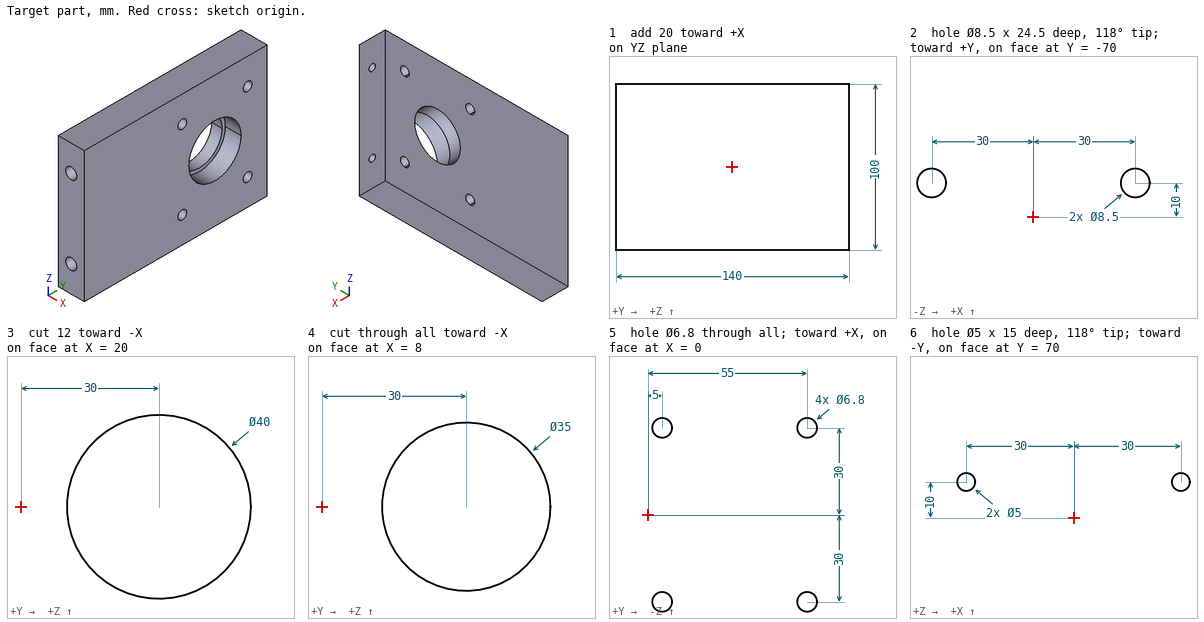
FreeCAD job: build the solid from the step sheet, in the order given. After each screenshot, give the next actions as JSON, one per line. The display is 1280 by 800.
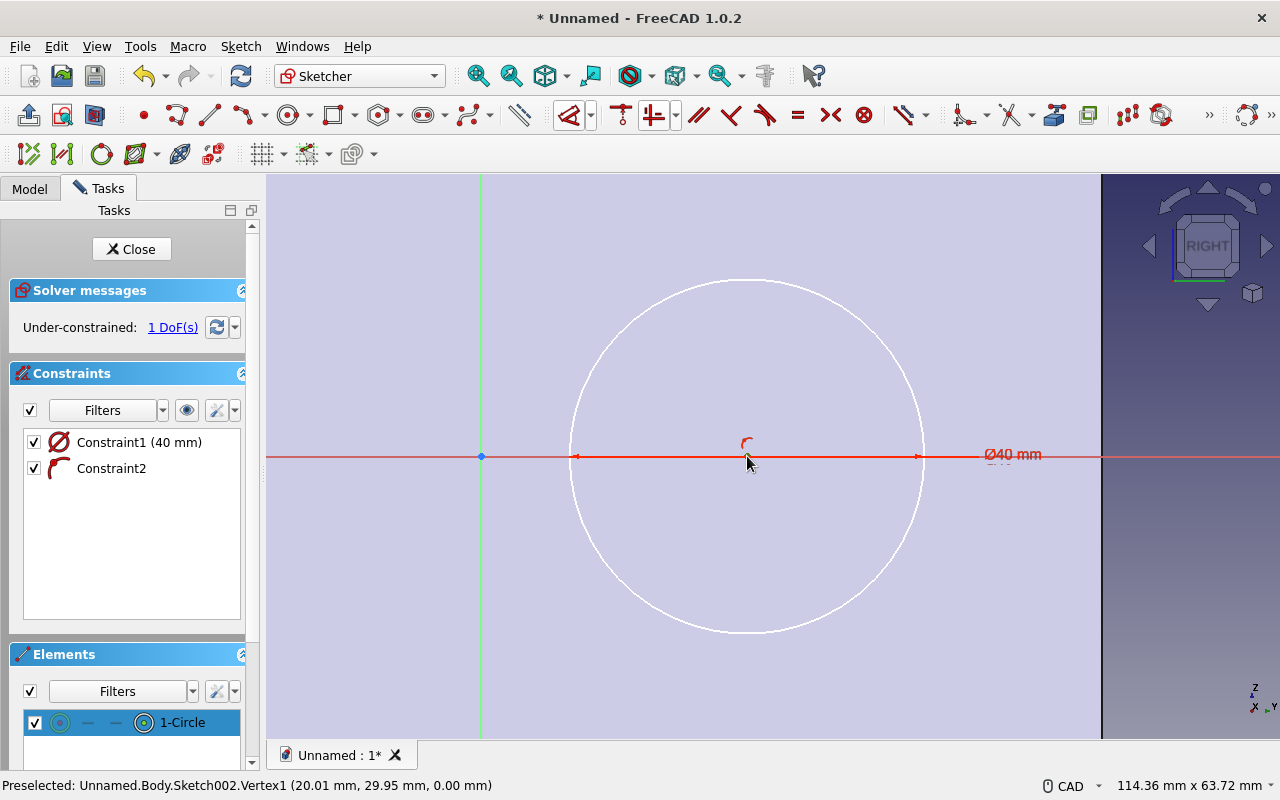
{"action": "left_click", "coordinate": [590, 116]}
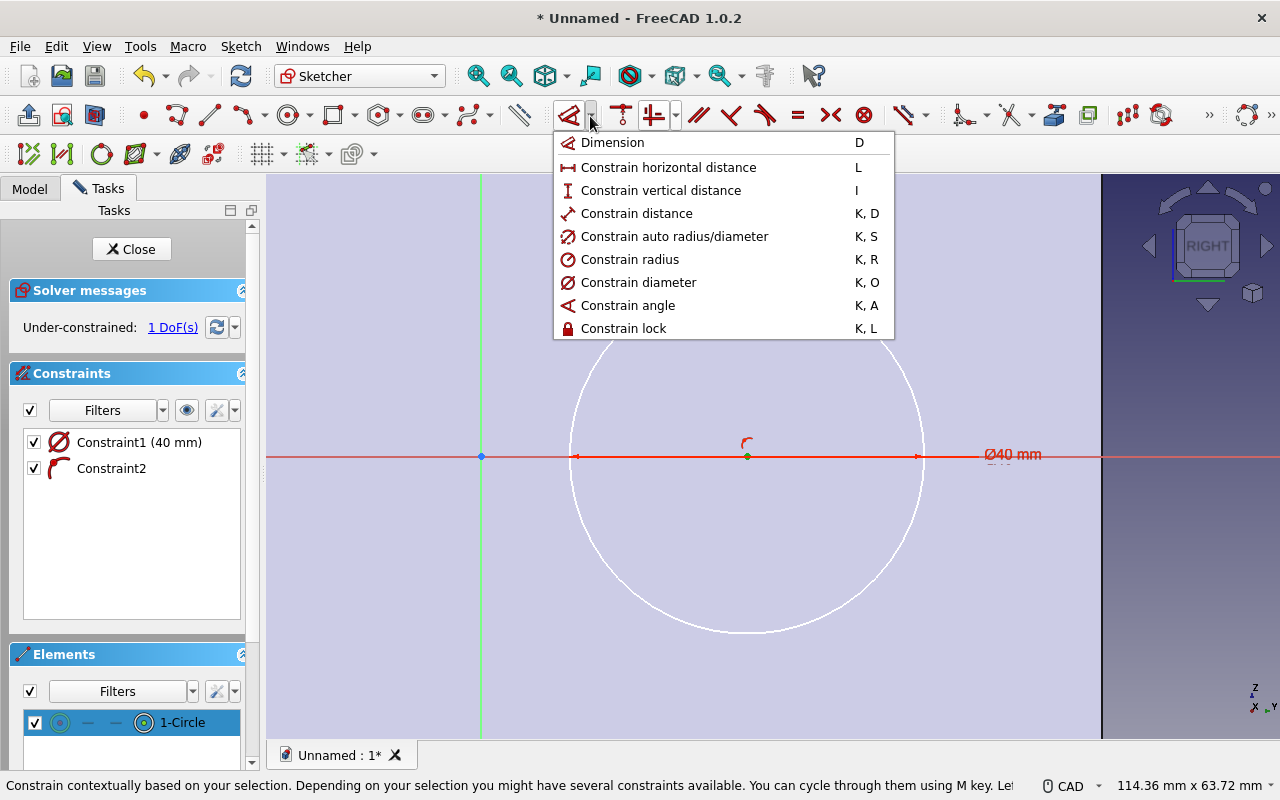
{"action": "left_click", "coordinate": [724, 168]}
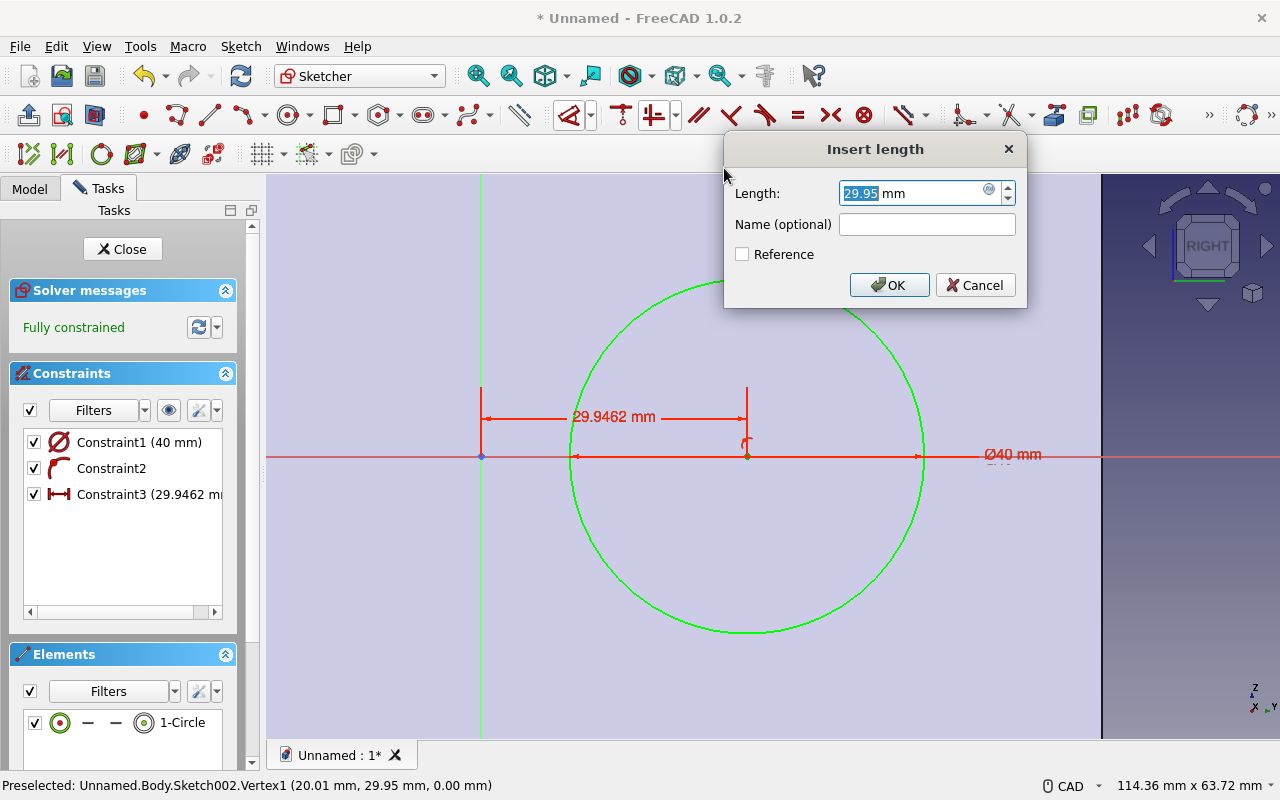
{"action": "type", "text": "30"}
{"action": "key", "text": "Return"}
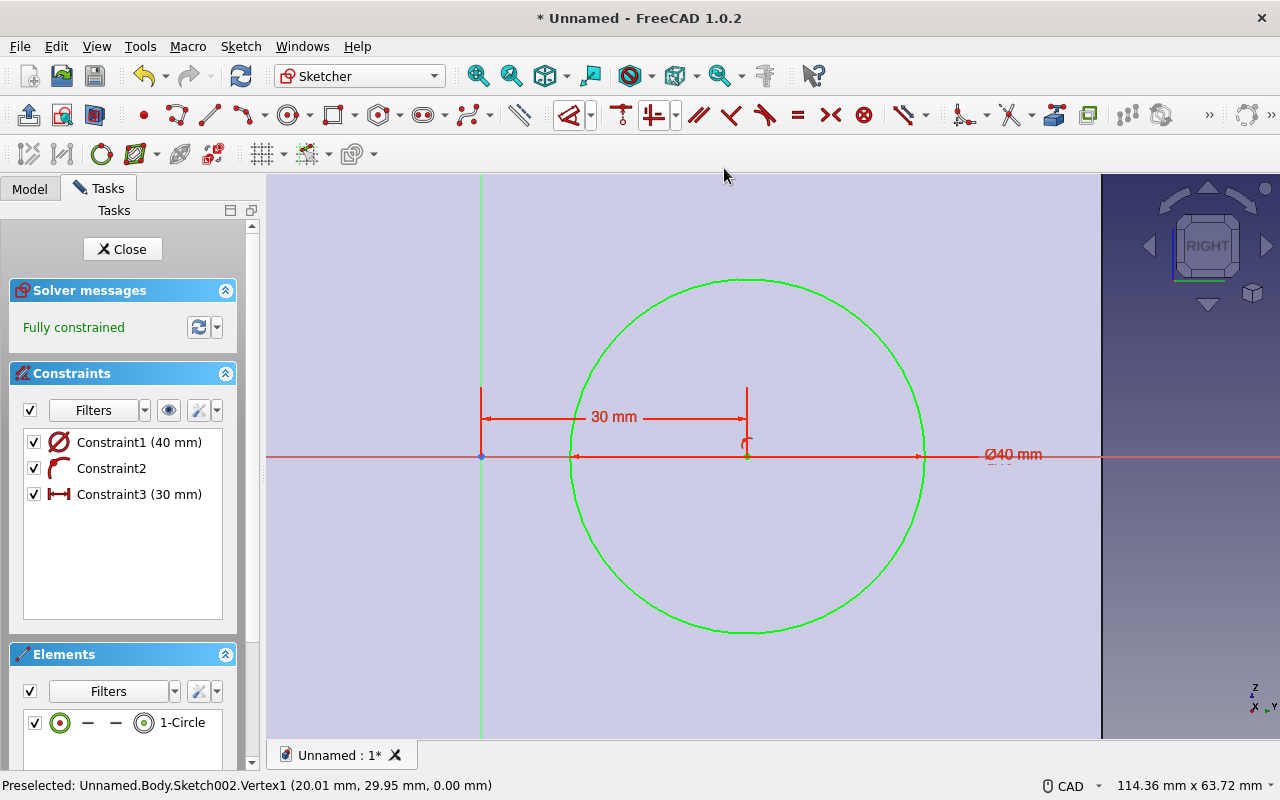
{"action": "left_click", "coordinate": [123, 249]}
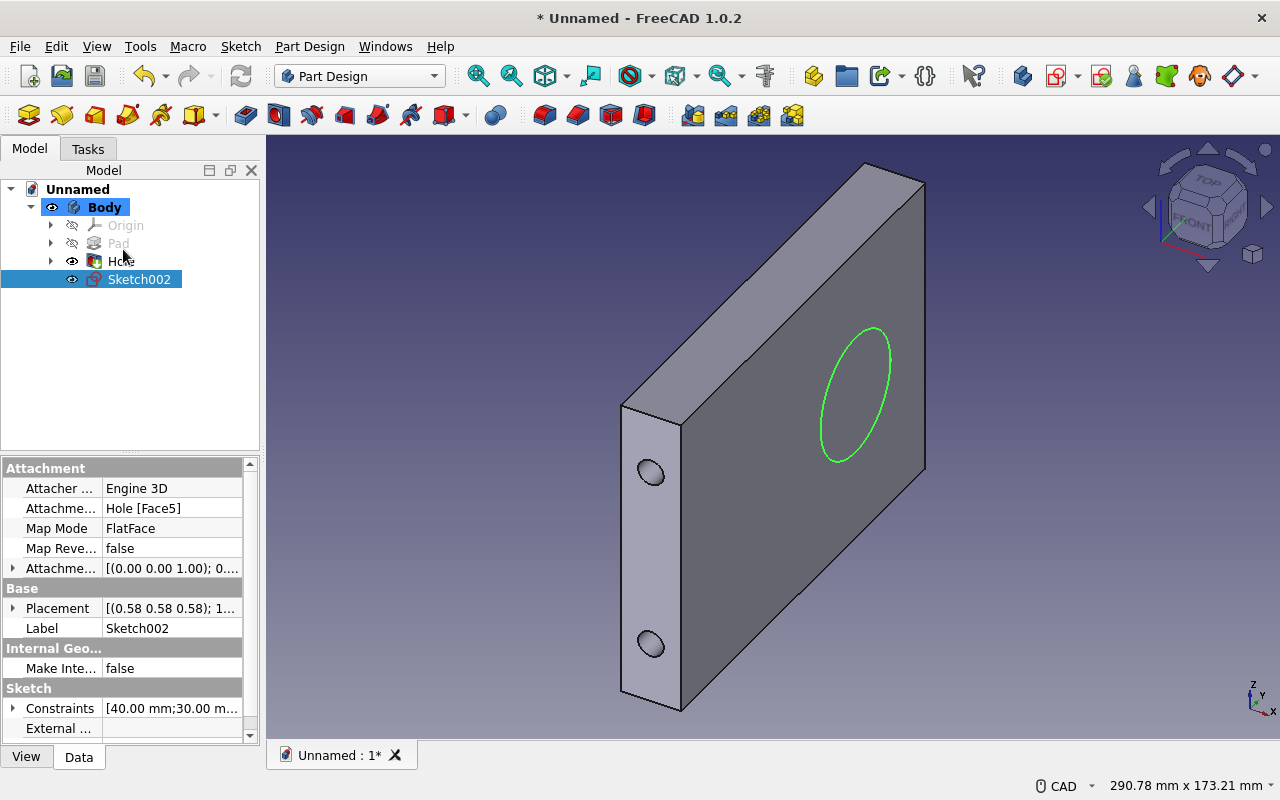
{"action": "left_click", "coordinate": [246, 116]}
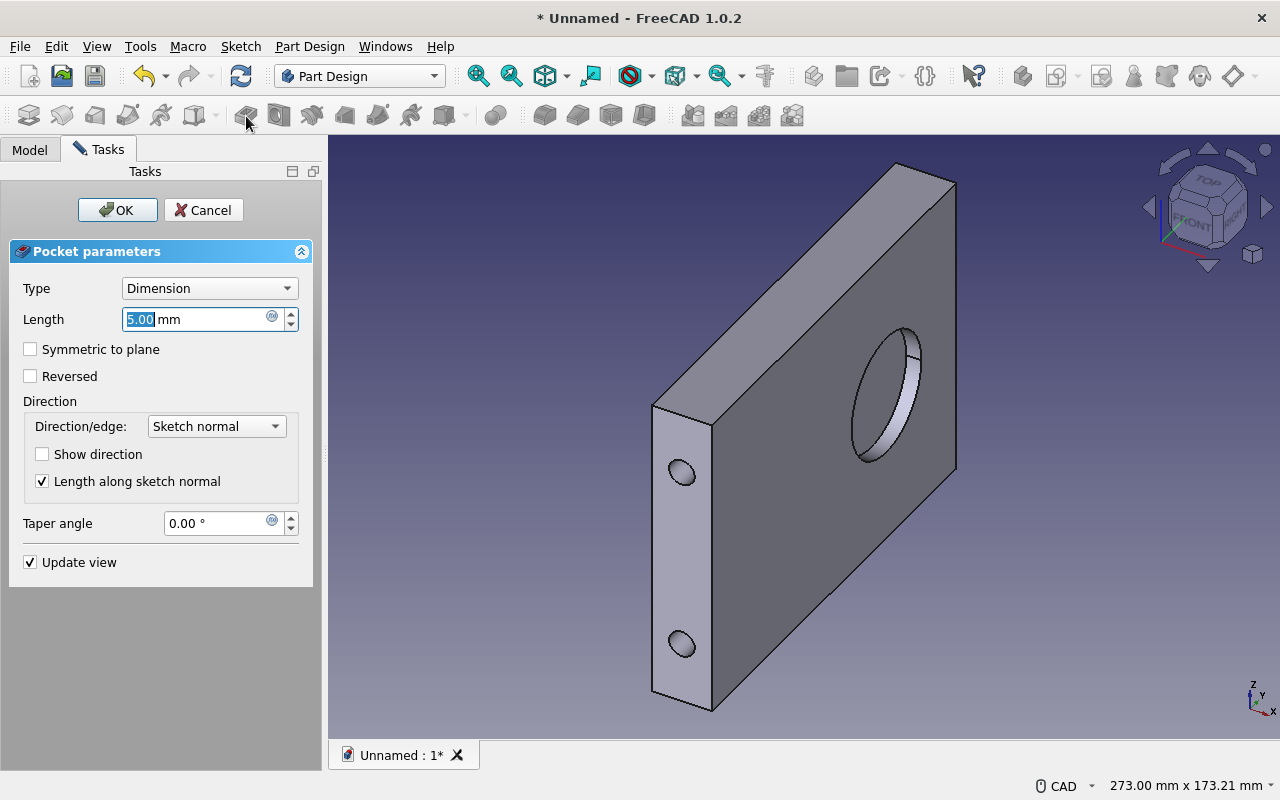
{"action": "type", "text": "12"}
{"action": "key", "text": "Tab"}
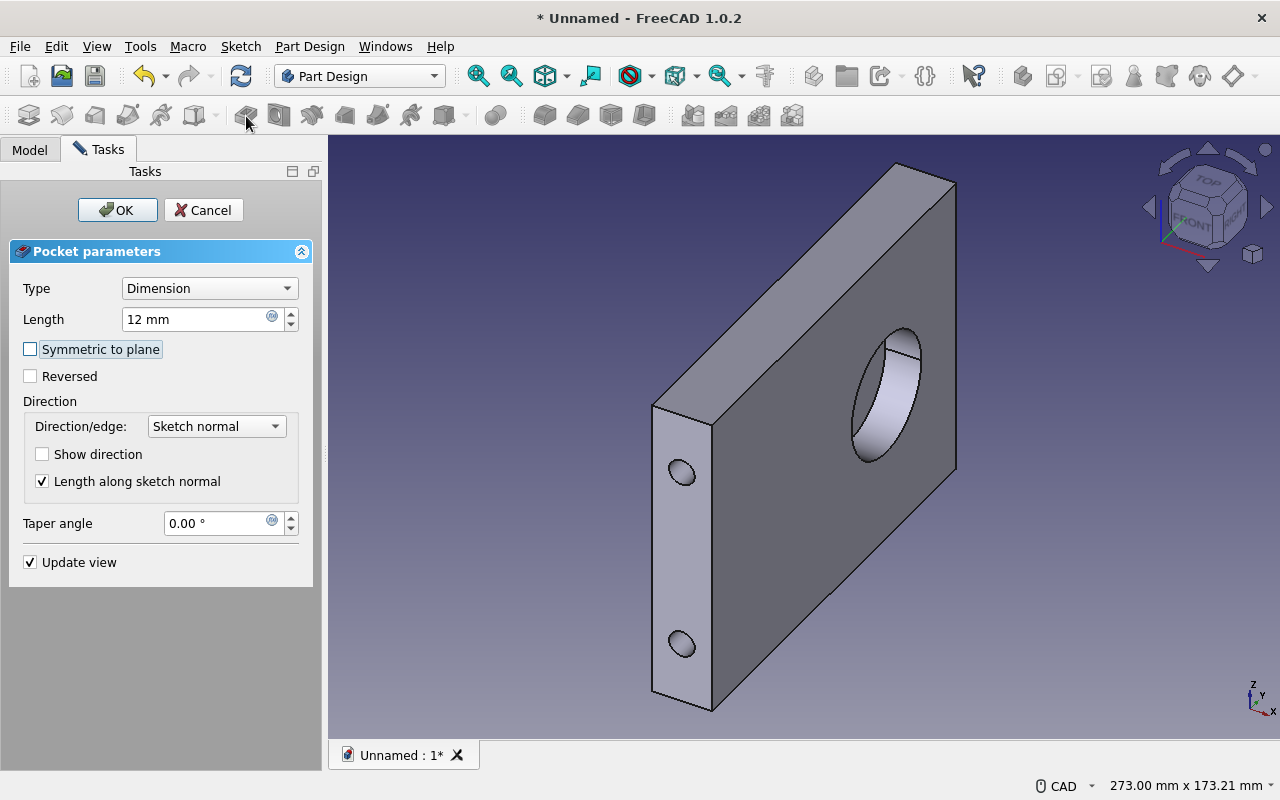
{"action": "left_click", "coordinate": [118, 210]}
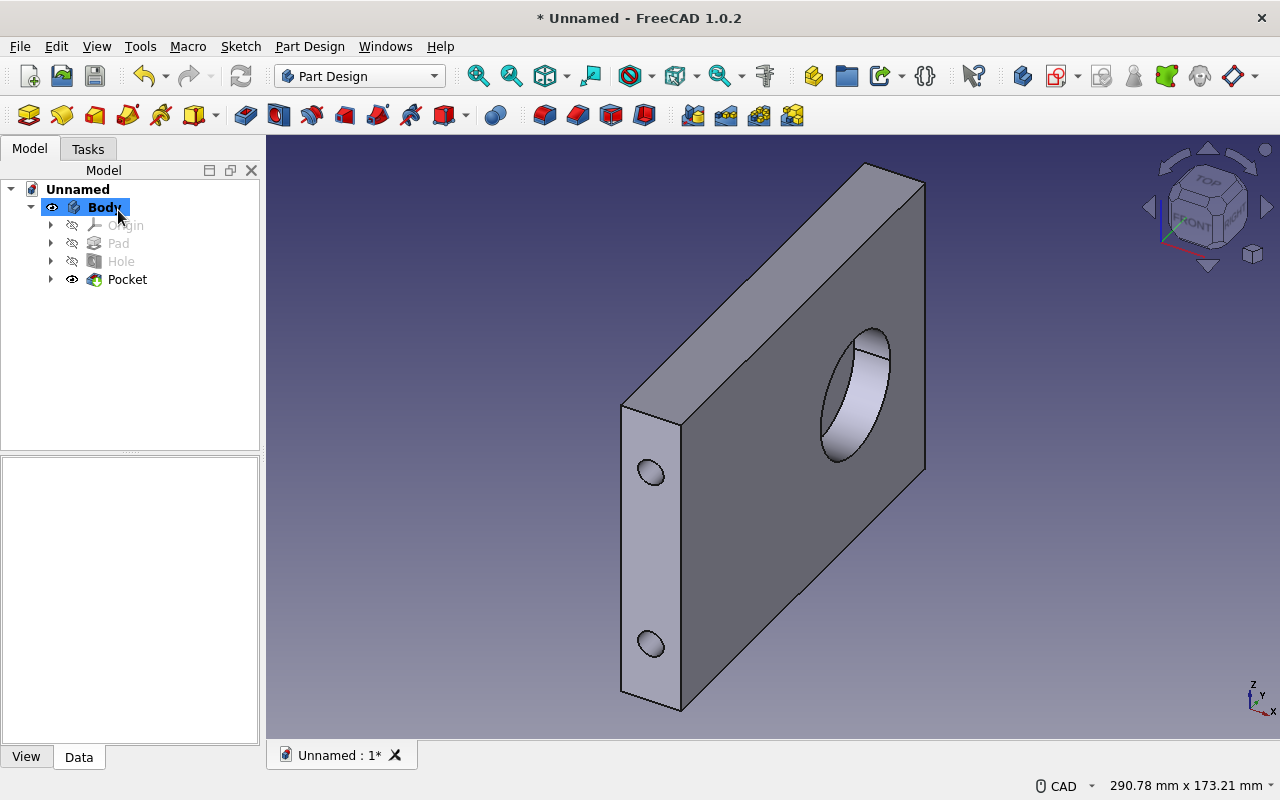
{"action": "key", "text": "0"}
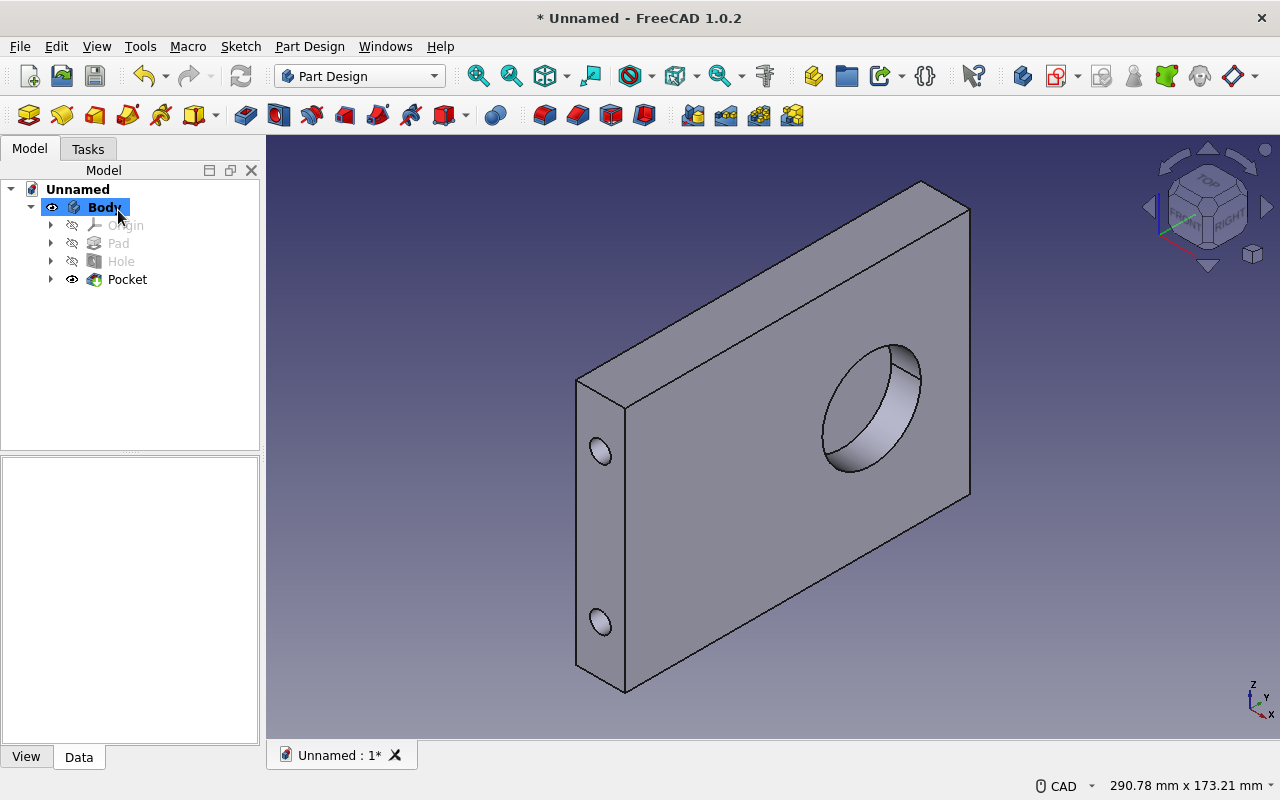
{"action": "left_click", "coordinate": [856, 382]}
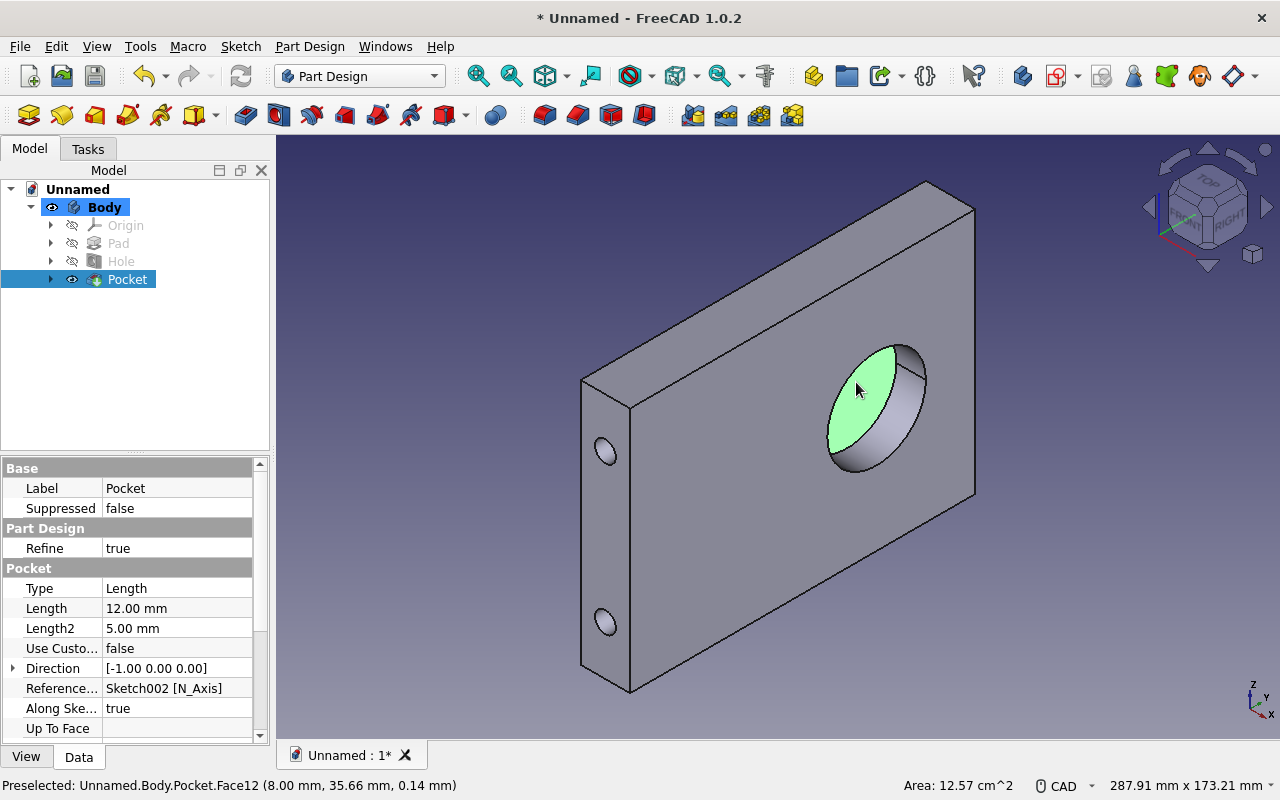
{"action": "left_click", "coordinate": [1056, 76]}